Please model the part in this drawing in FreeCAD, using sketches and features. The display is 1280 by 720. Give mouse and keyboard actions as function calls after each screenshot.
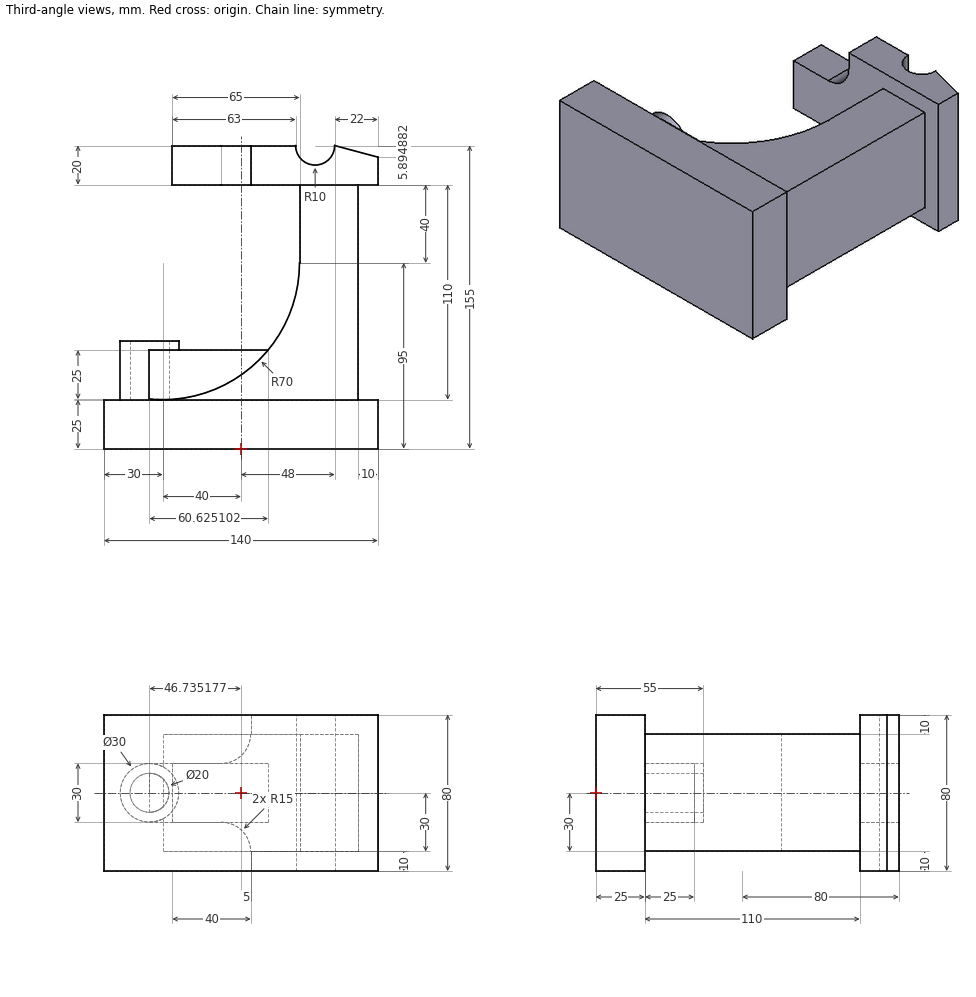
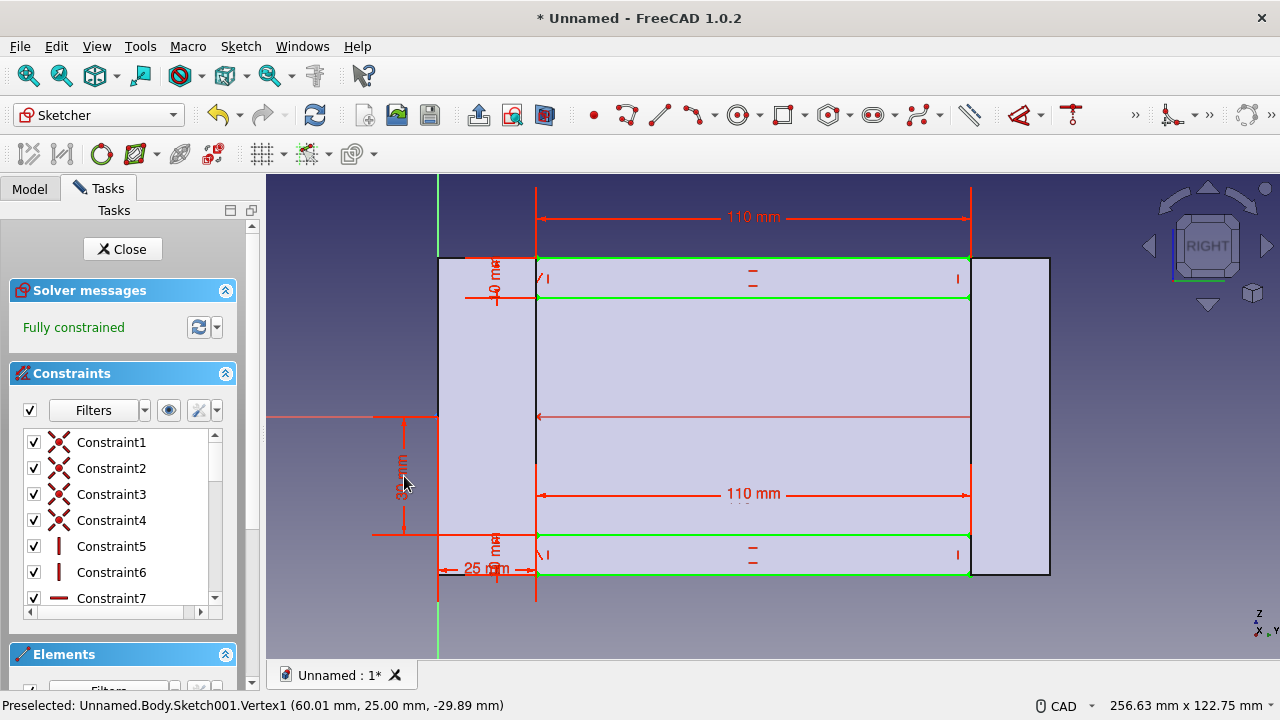
click(123, 249)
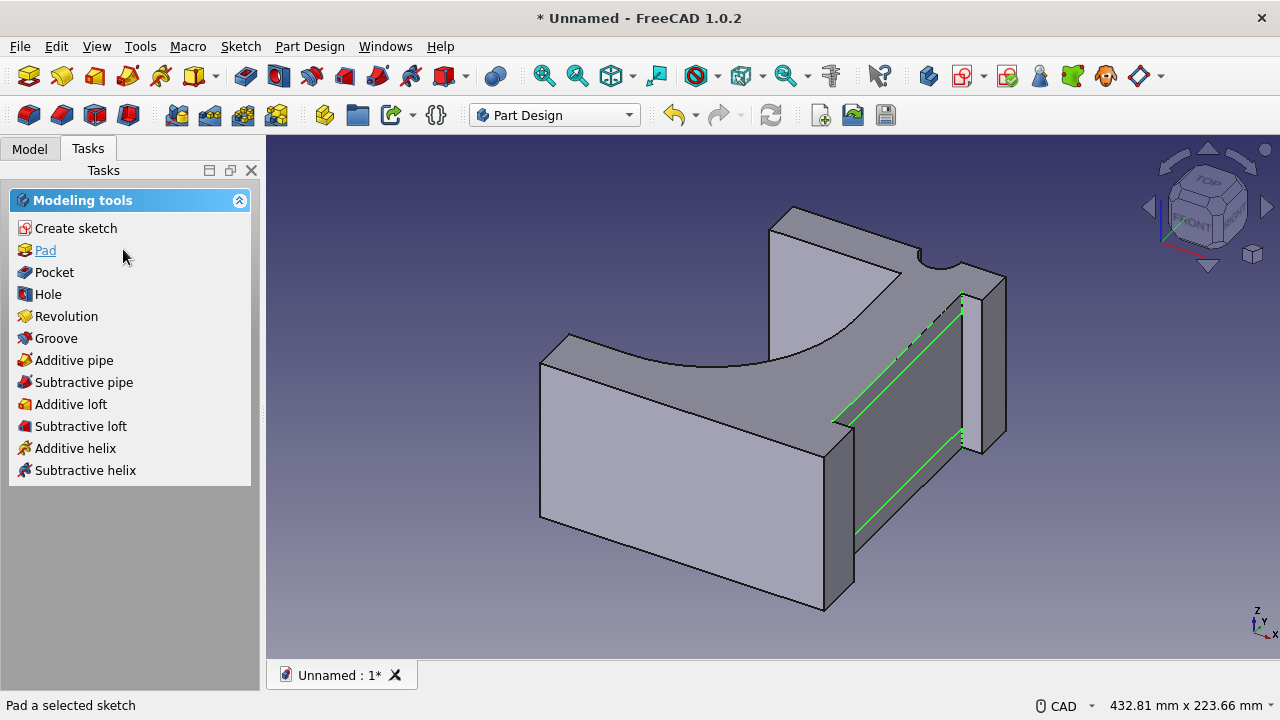
click(246, 76)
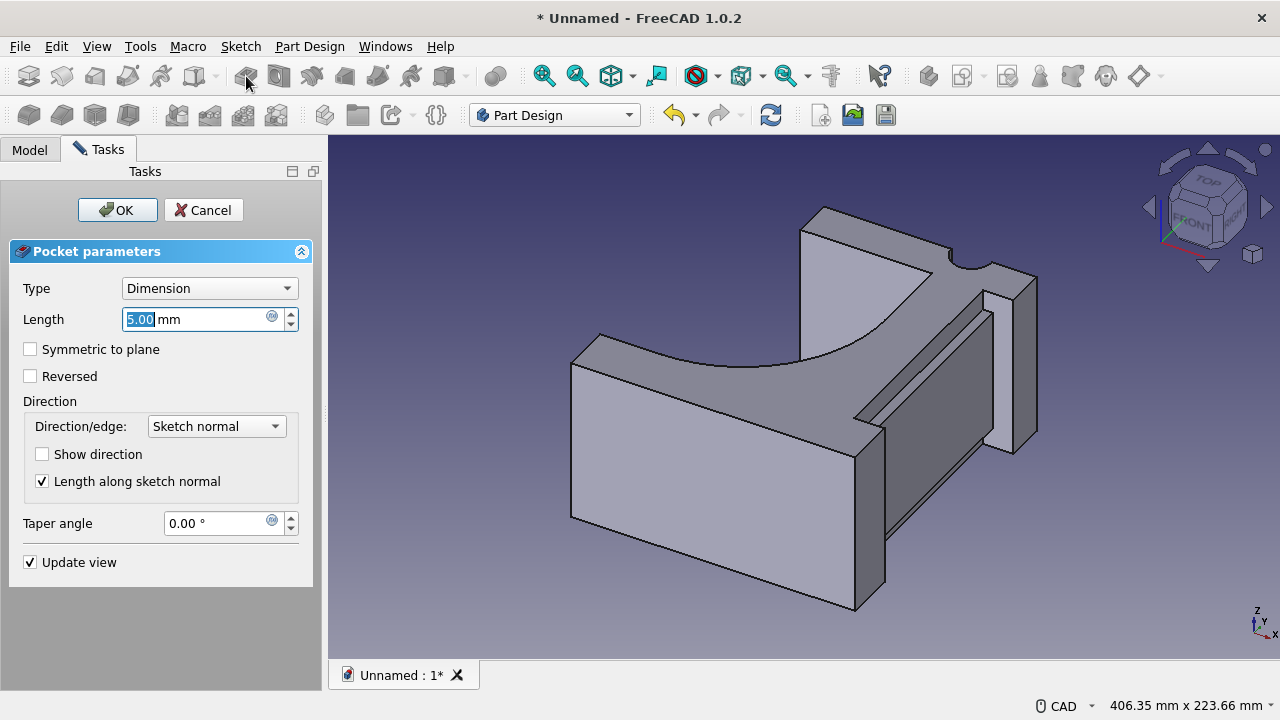
click(210, 288)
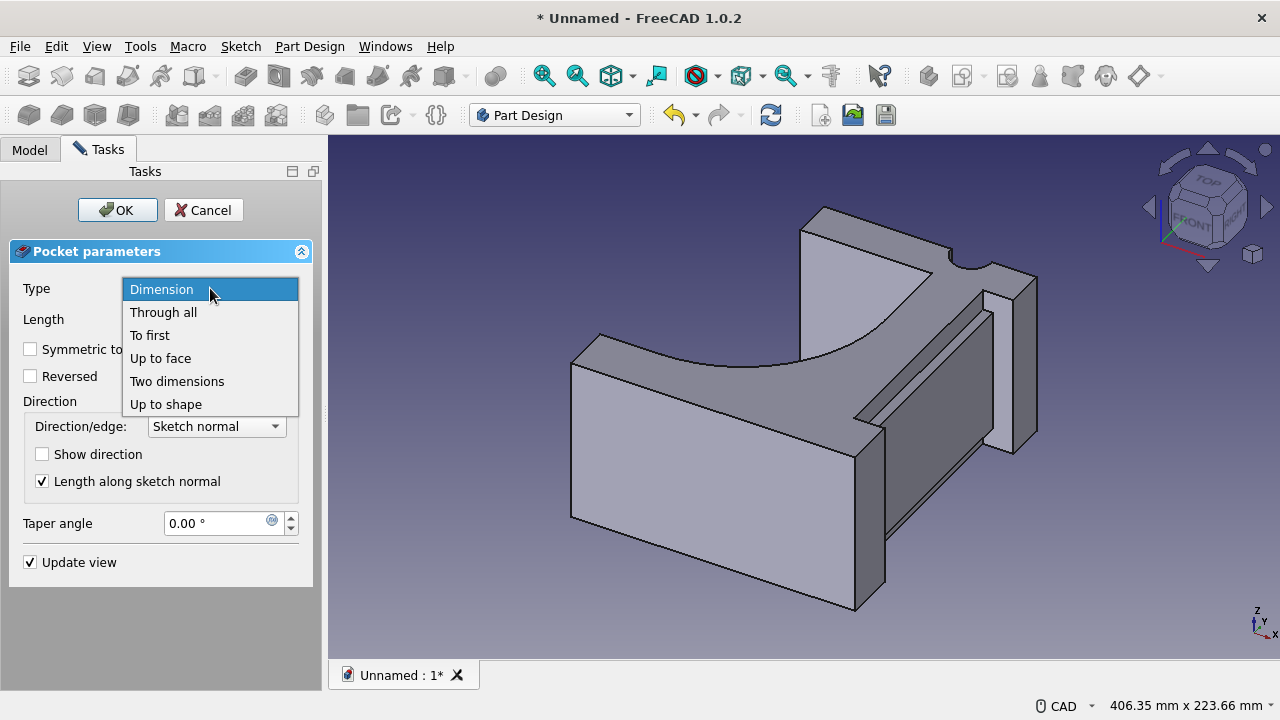
click(208, 312)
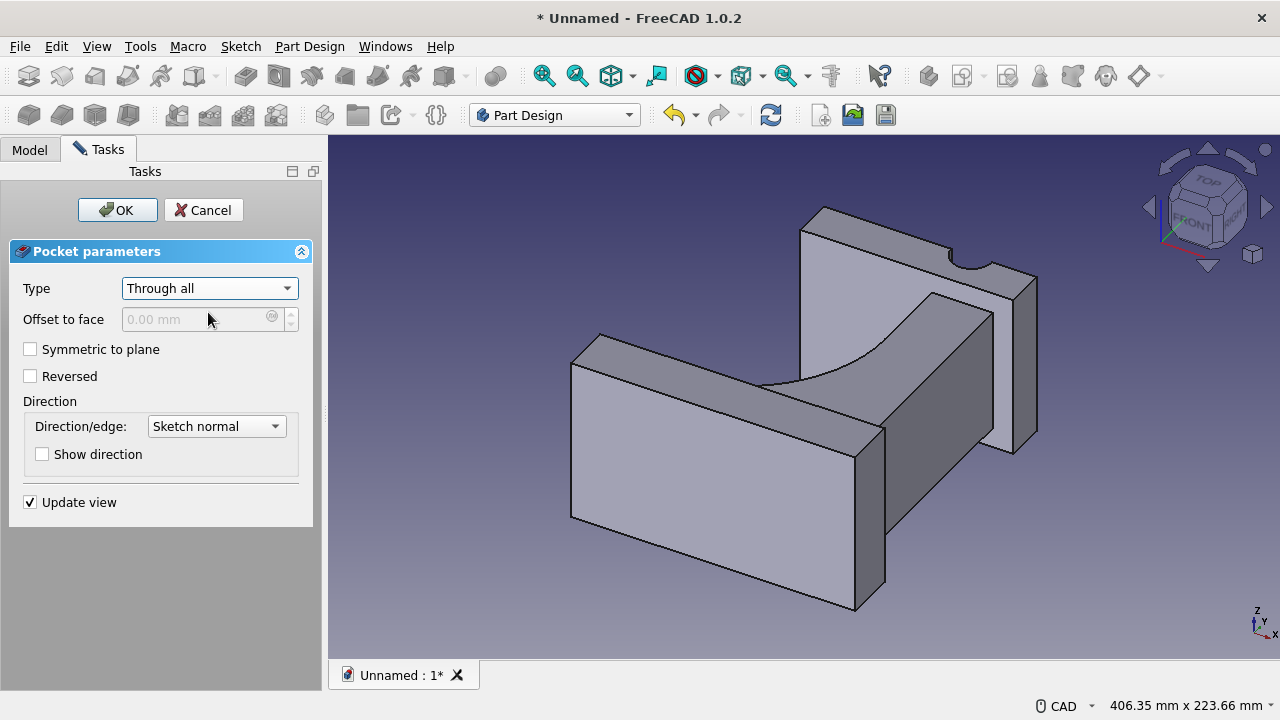
click(118, 210)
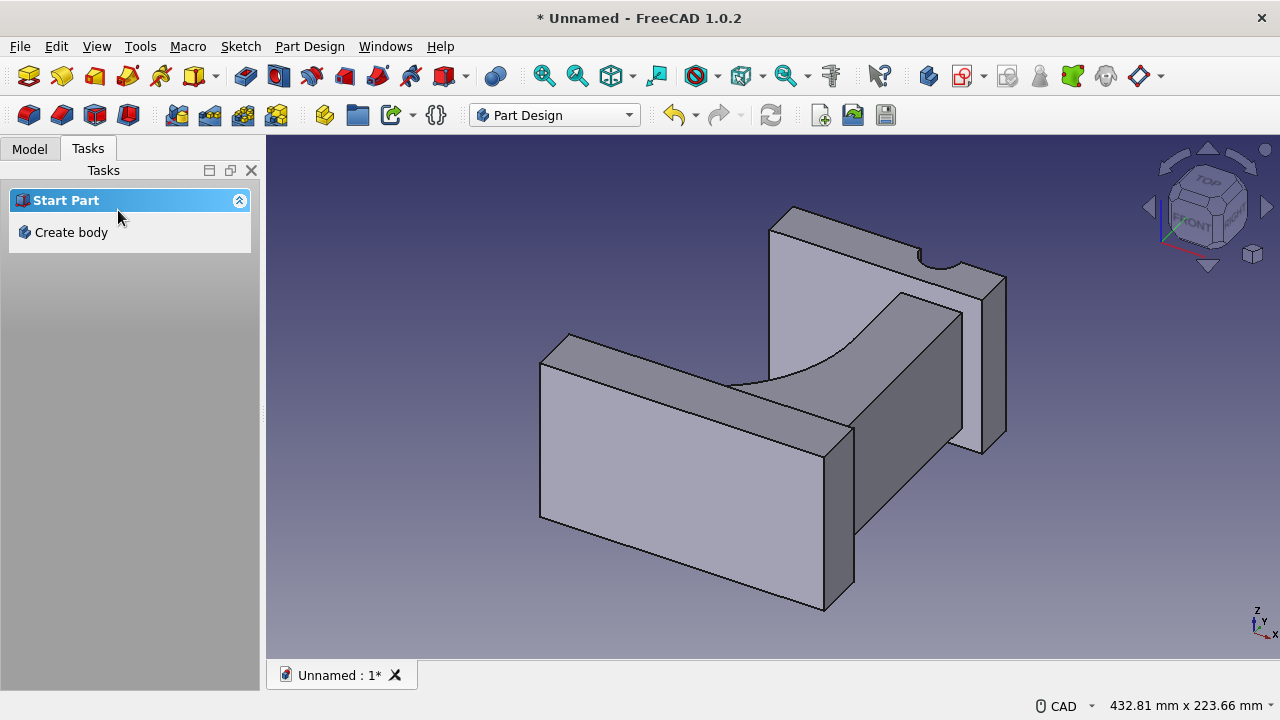
key(4)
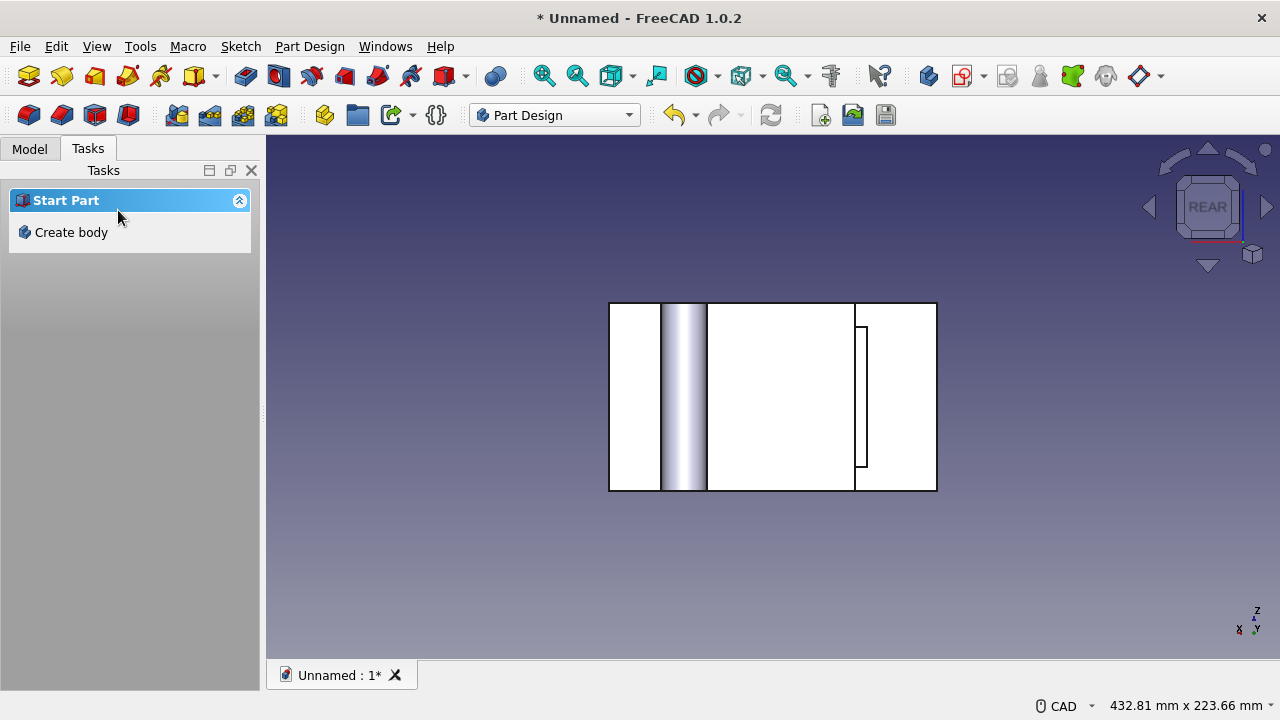
click(545, 76)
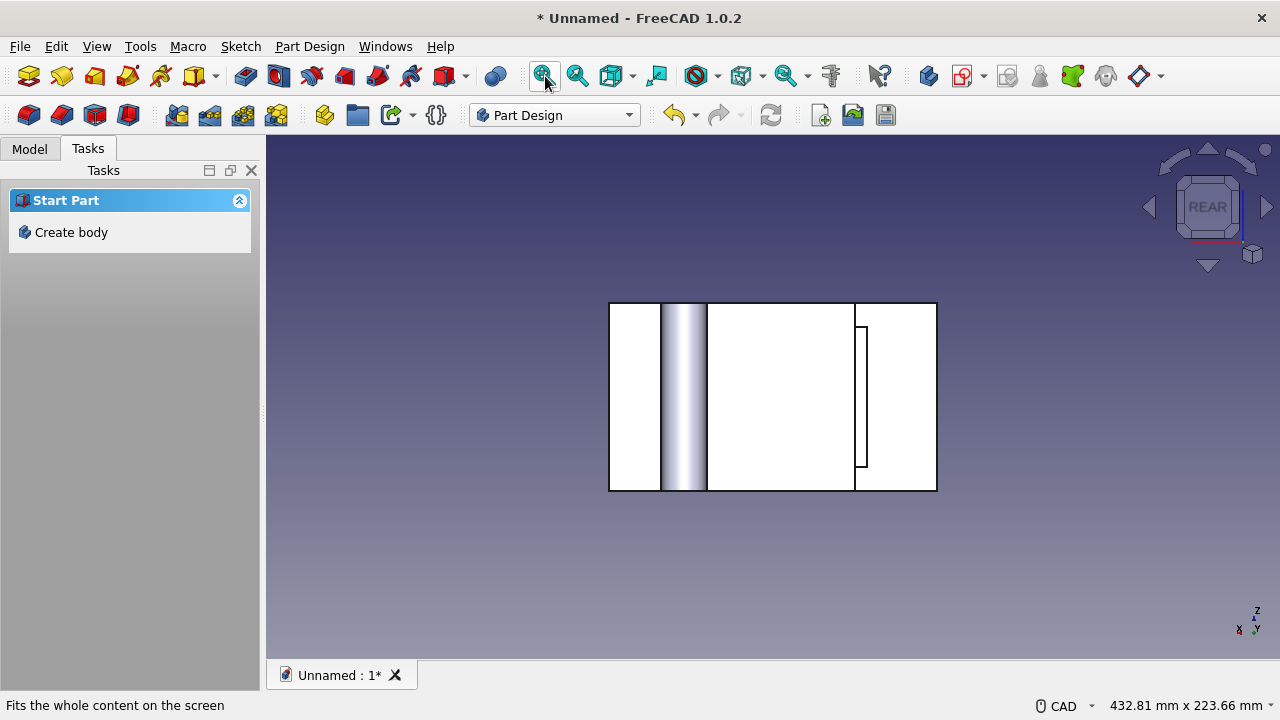
click(781, 396)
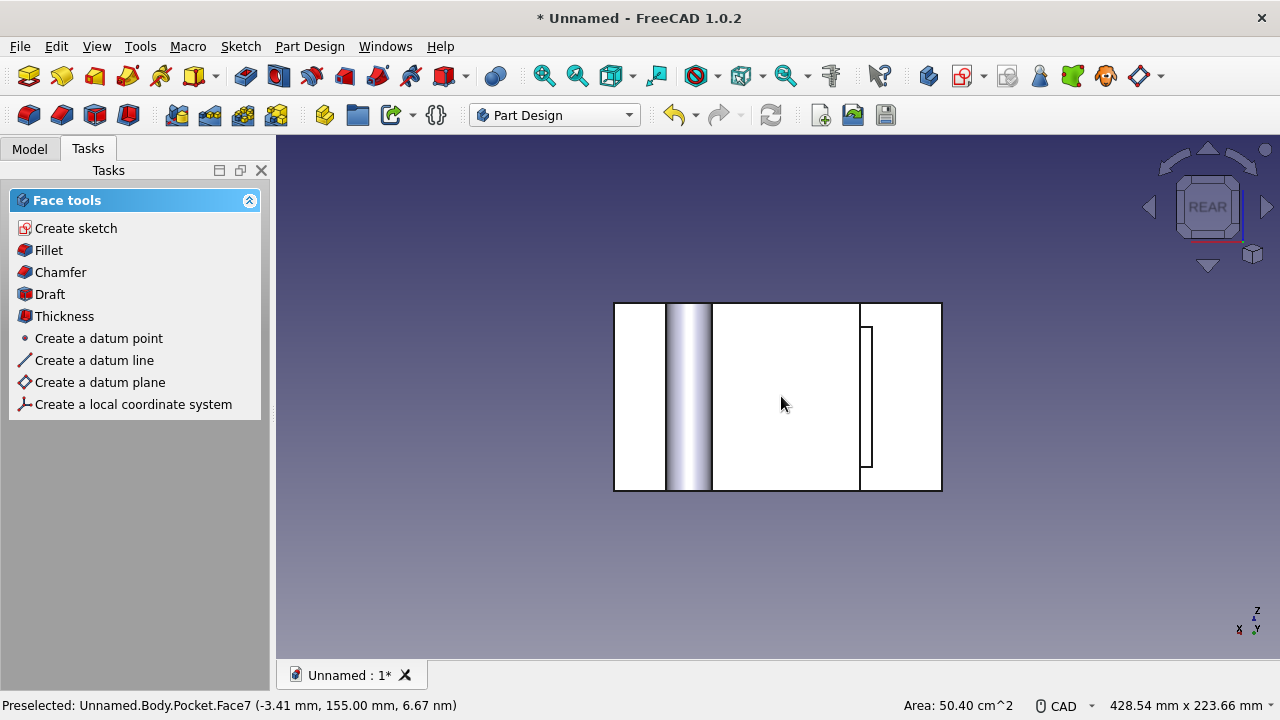
click(962, 76)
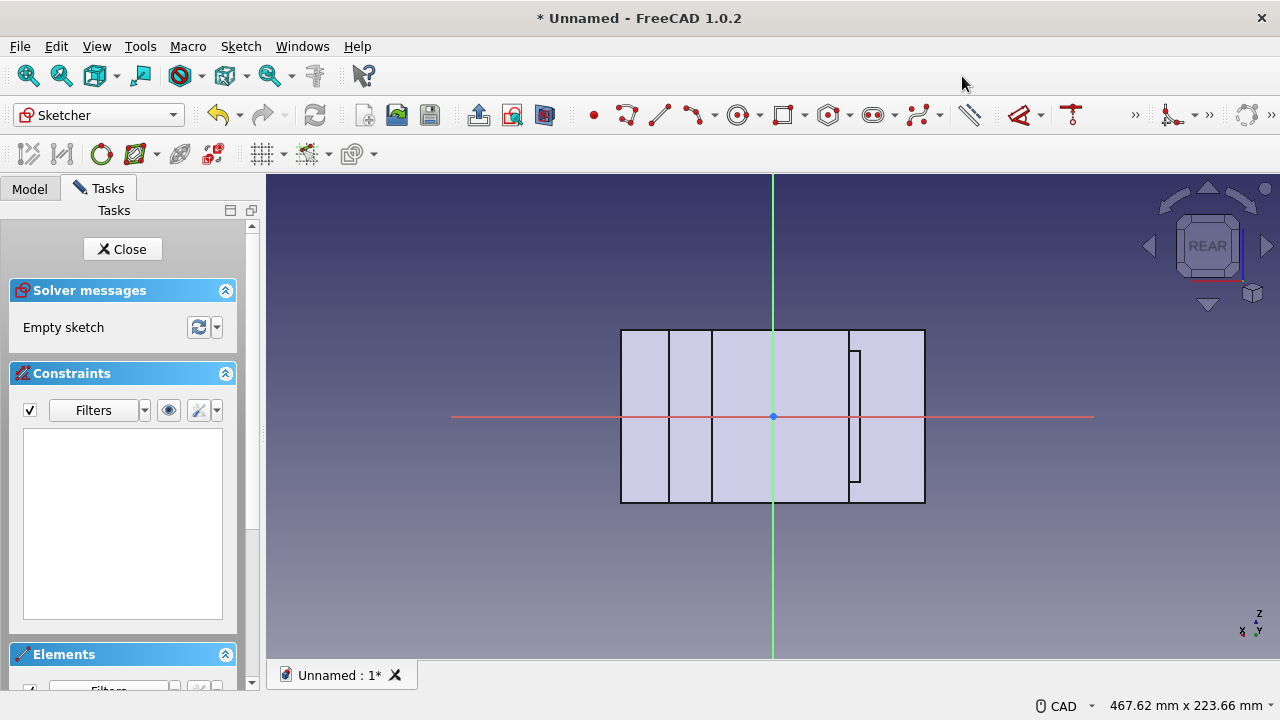
scroll(928, 417, up, 3)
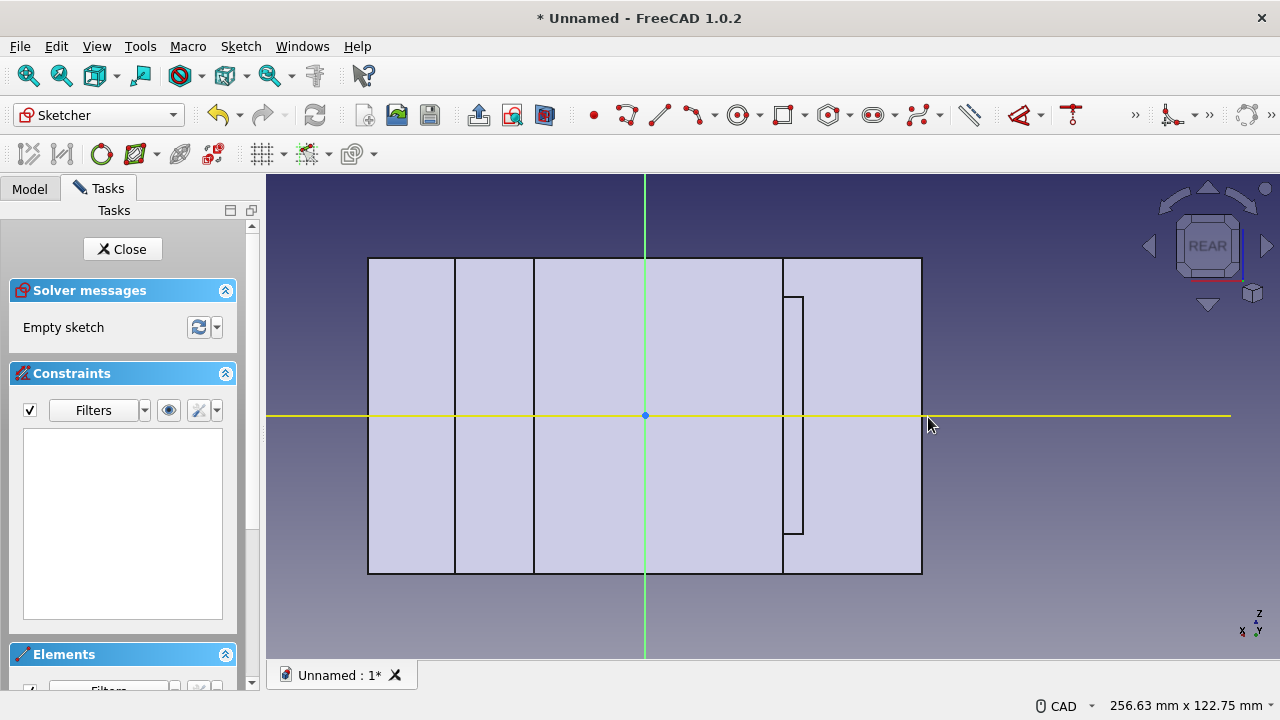
click(627, 116)